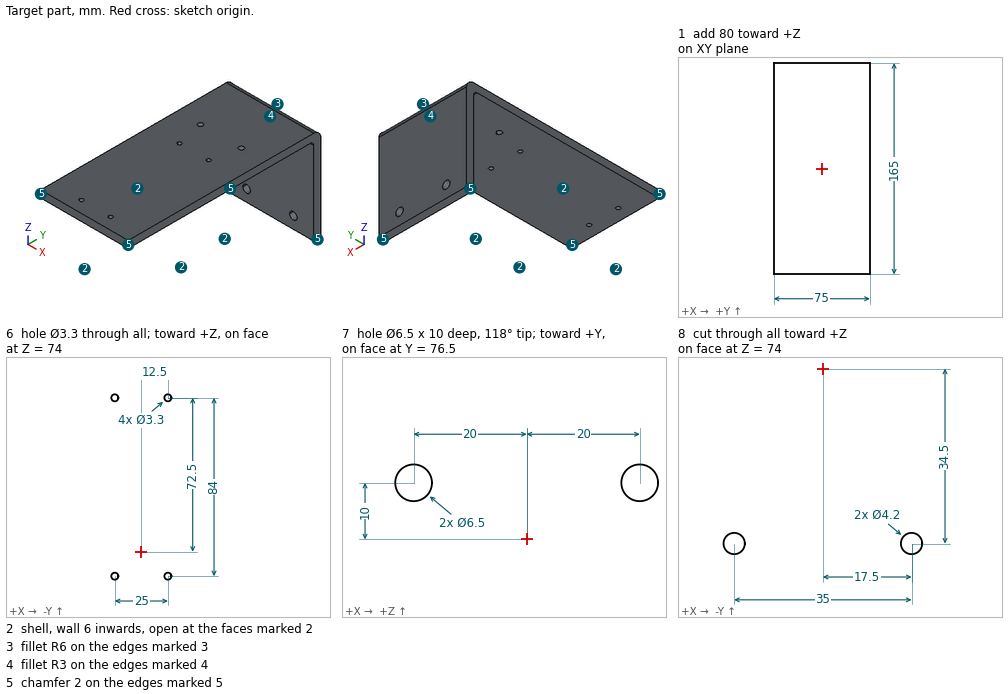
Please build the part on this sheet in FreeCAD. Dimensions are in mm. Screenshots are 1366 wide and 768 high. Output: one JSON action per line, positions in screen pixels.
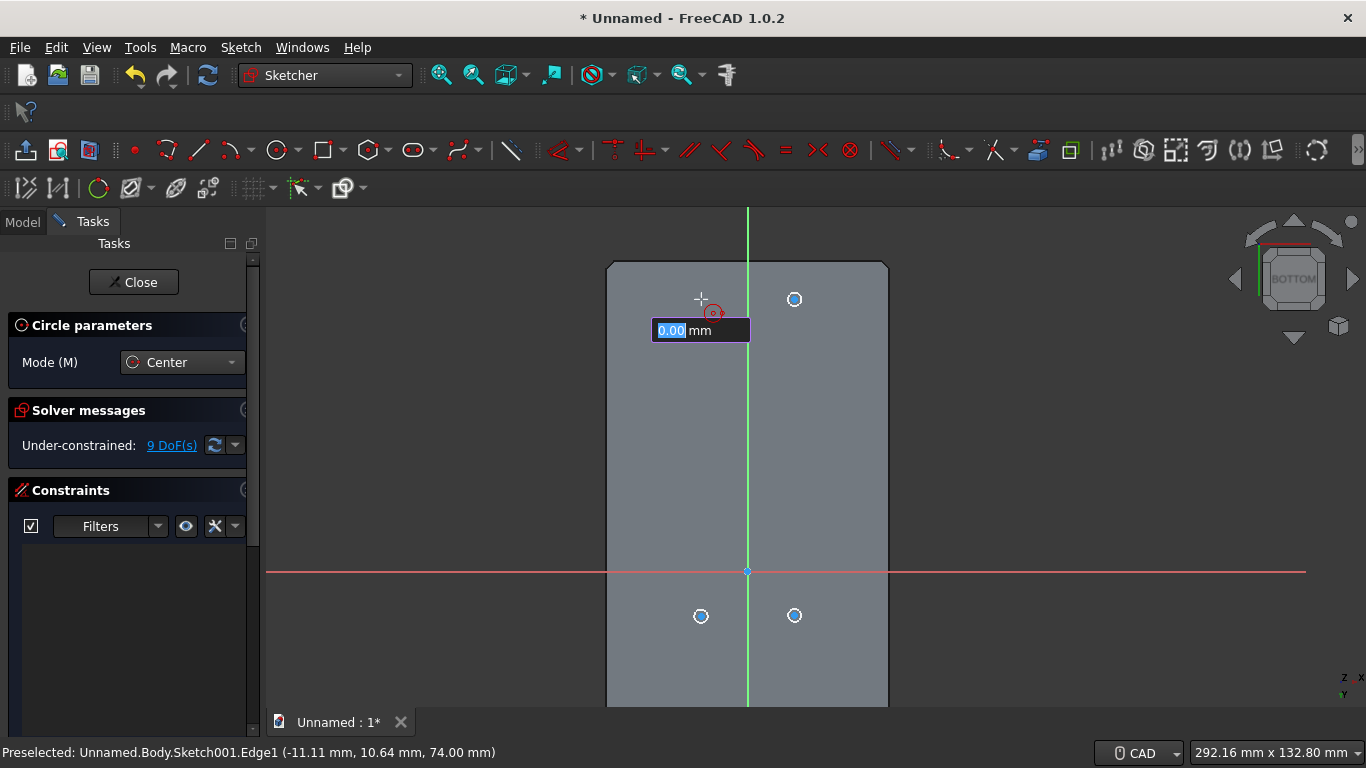
{"action": "scroll", "coordinate": [705, 294], "scroll_direction": "up", "scroll_amount": 5}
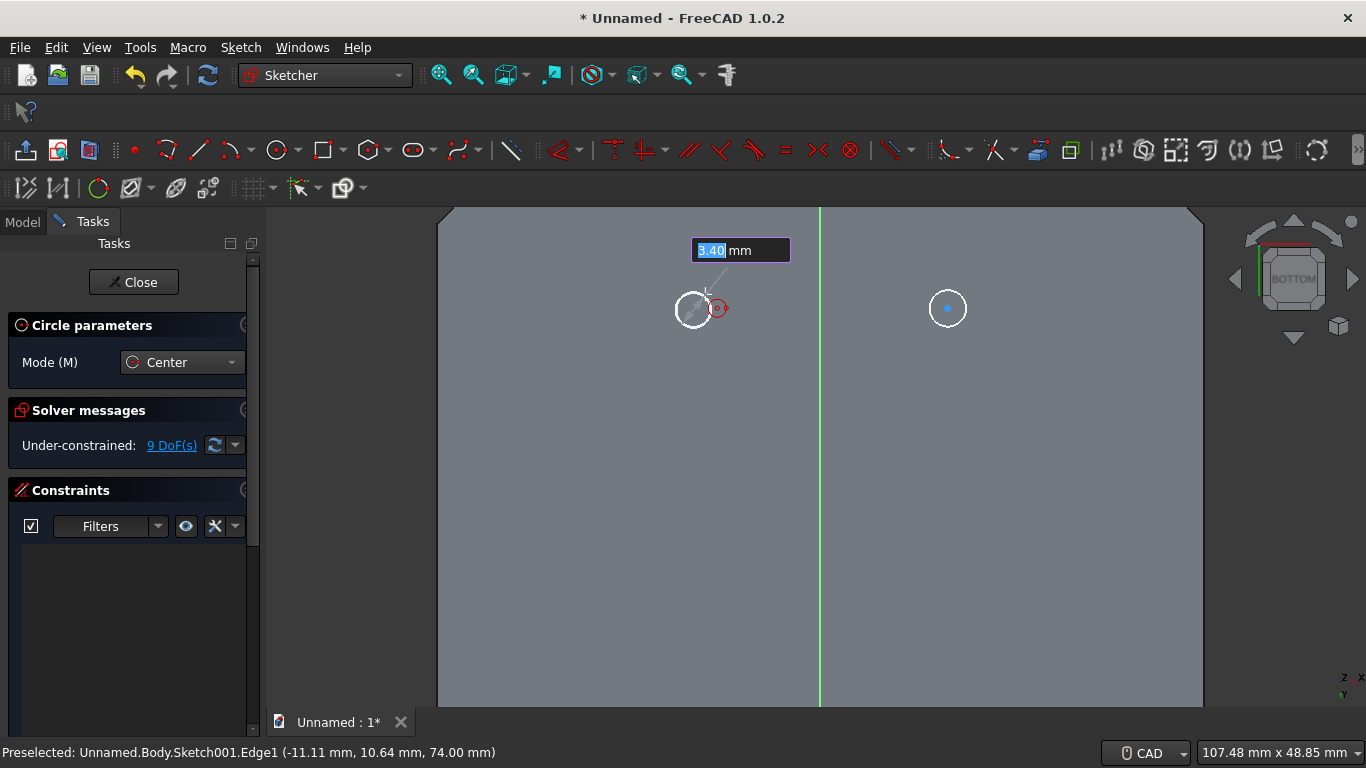
{"action": "left_click", "coordinate": [704, 294]}
{"action": "key", "text": "Escape"}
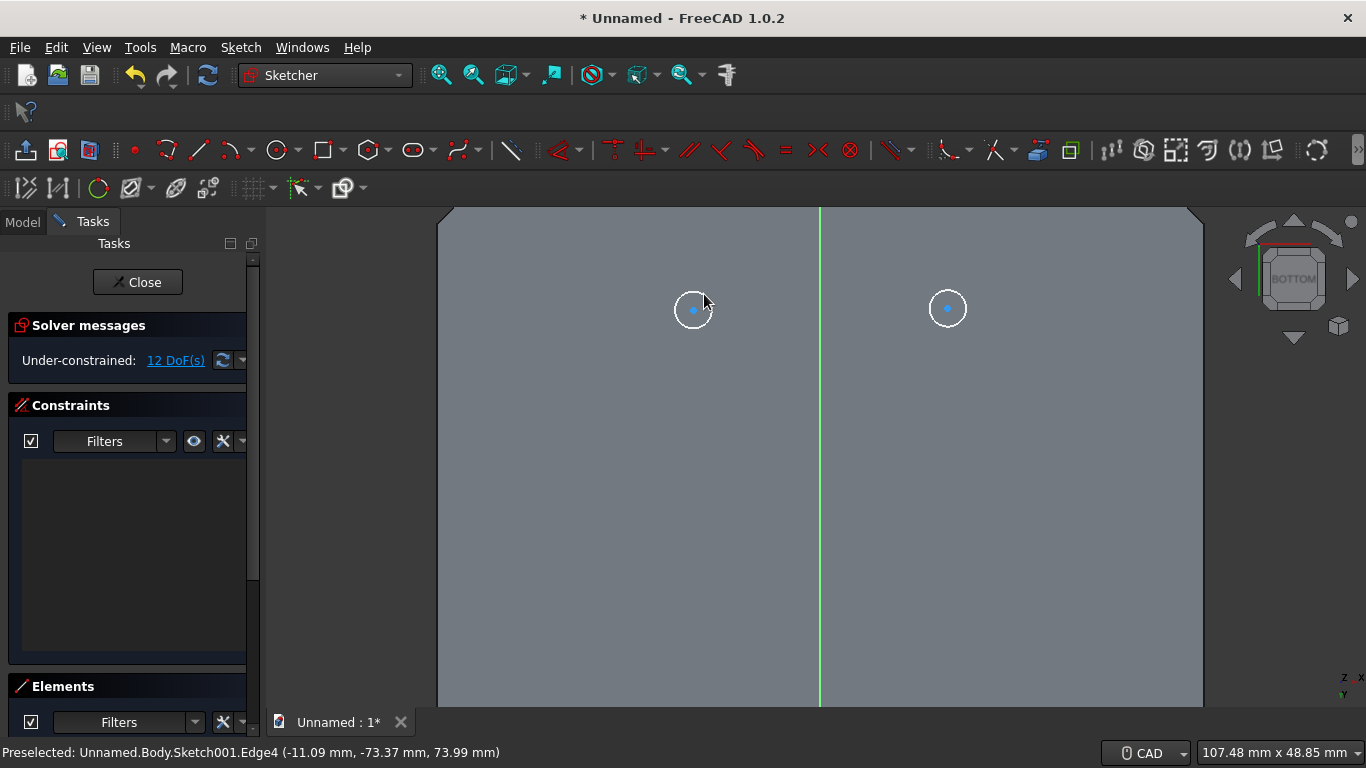
{"action": "left_click", "coordinate": [961, 296]}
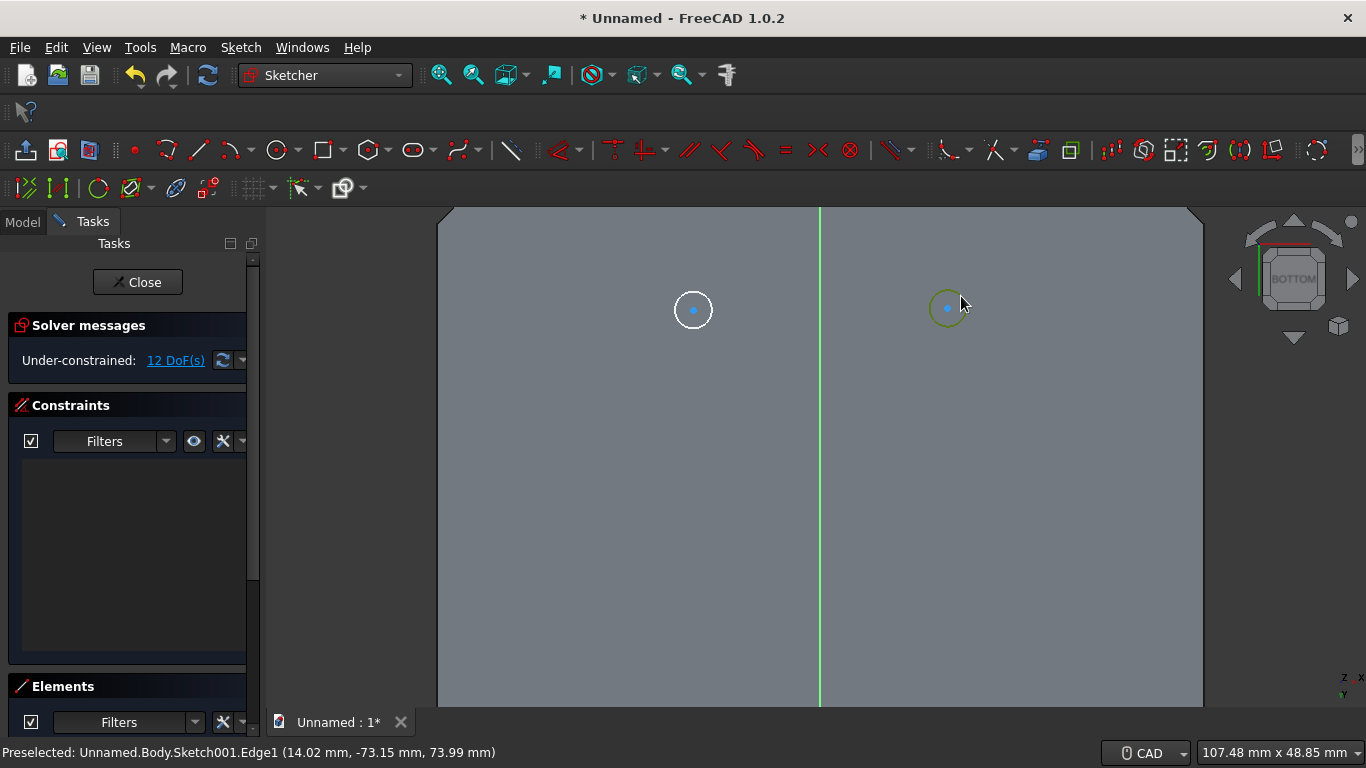
{"action": "scroll", "coordinate": [705, 295], "scroll_direction": "down", "scroll_amount": 5}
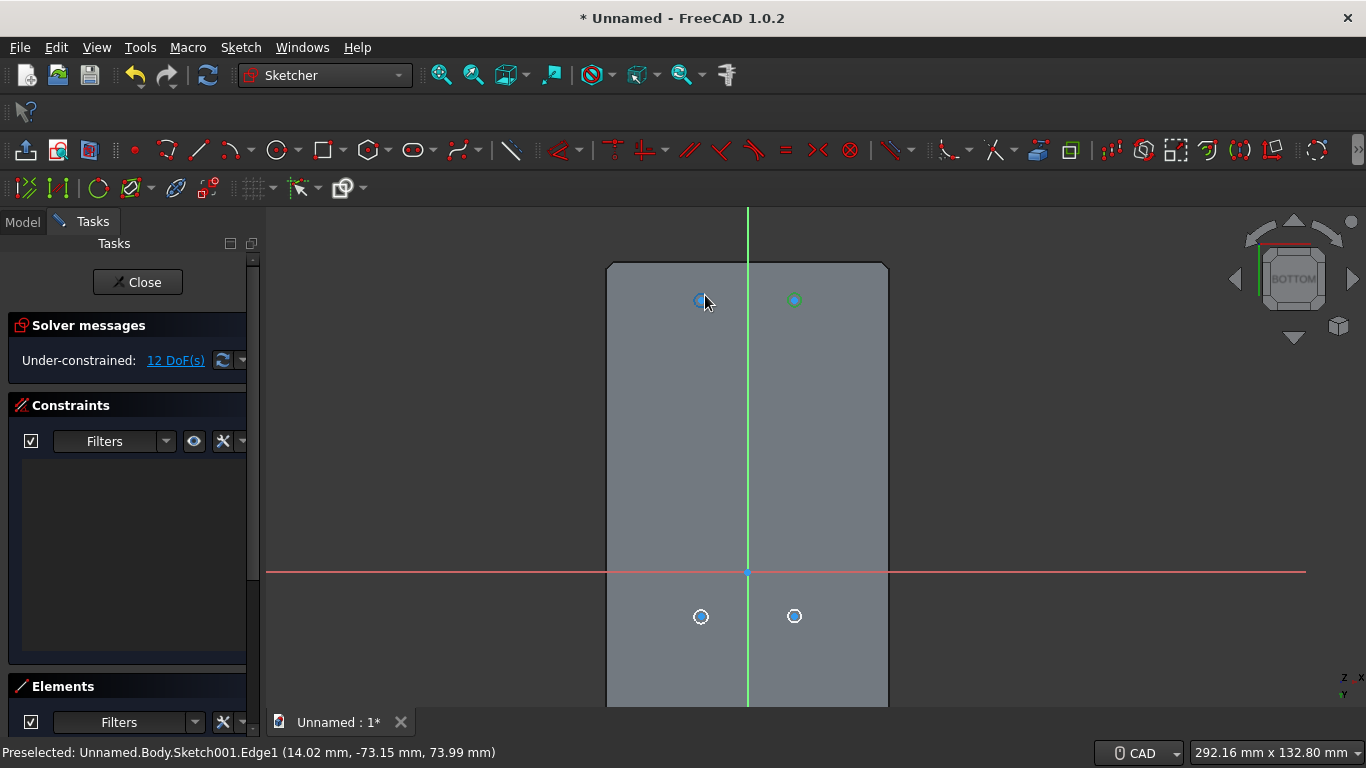
{"action": "scroll", "coordinate": [799, 612], "scroll_direction": "up", "scroll_amount": 4}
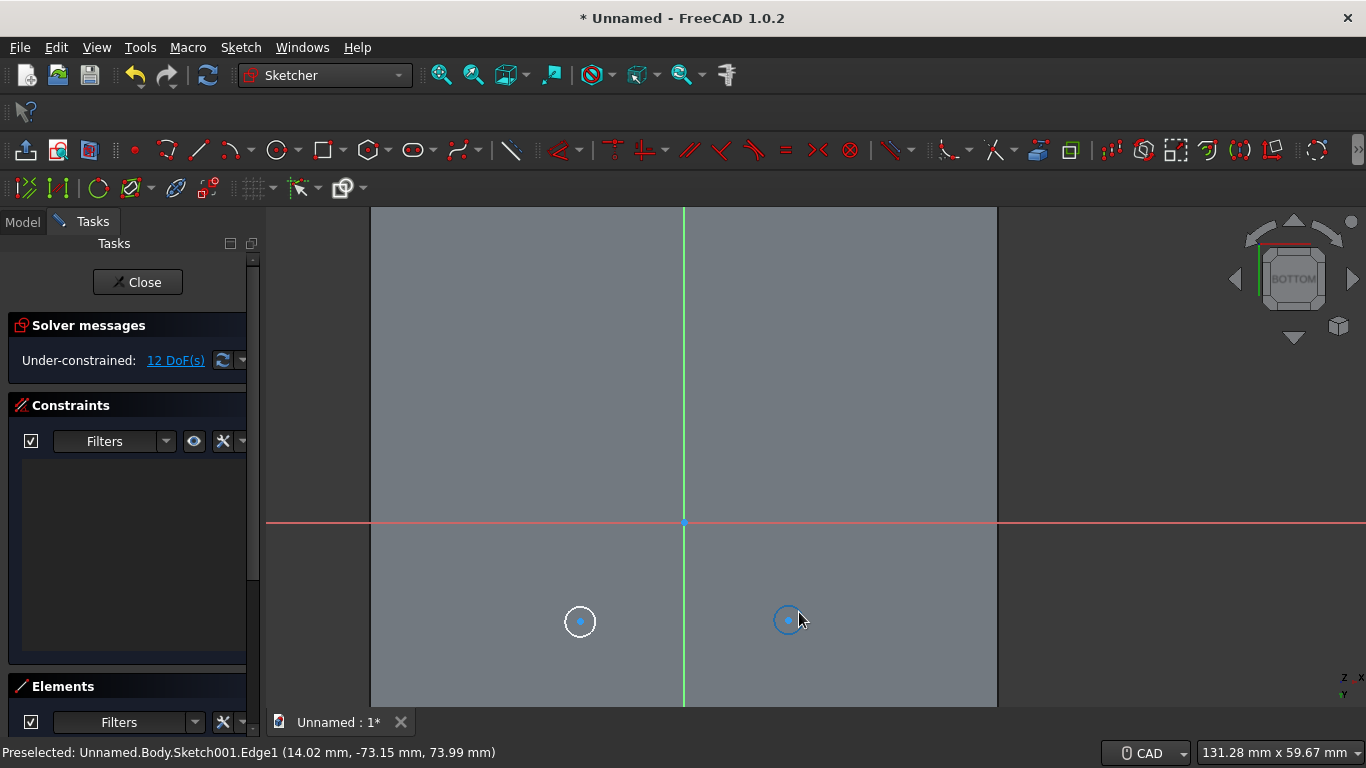
{"action": "left_click", "coordinate": [799, 610]}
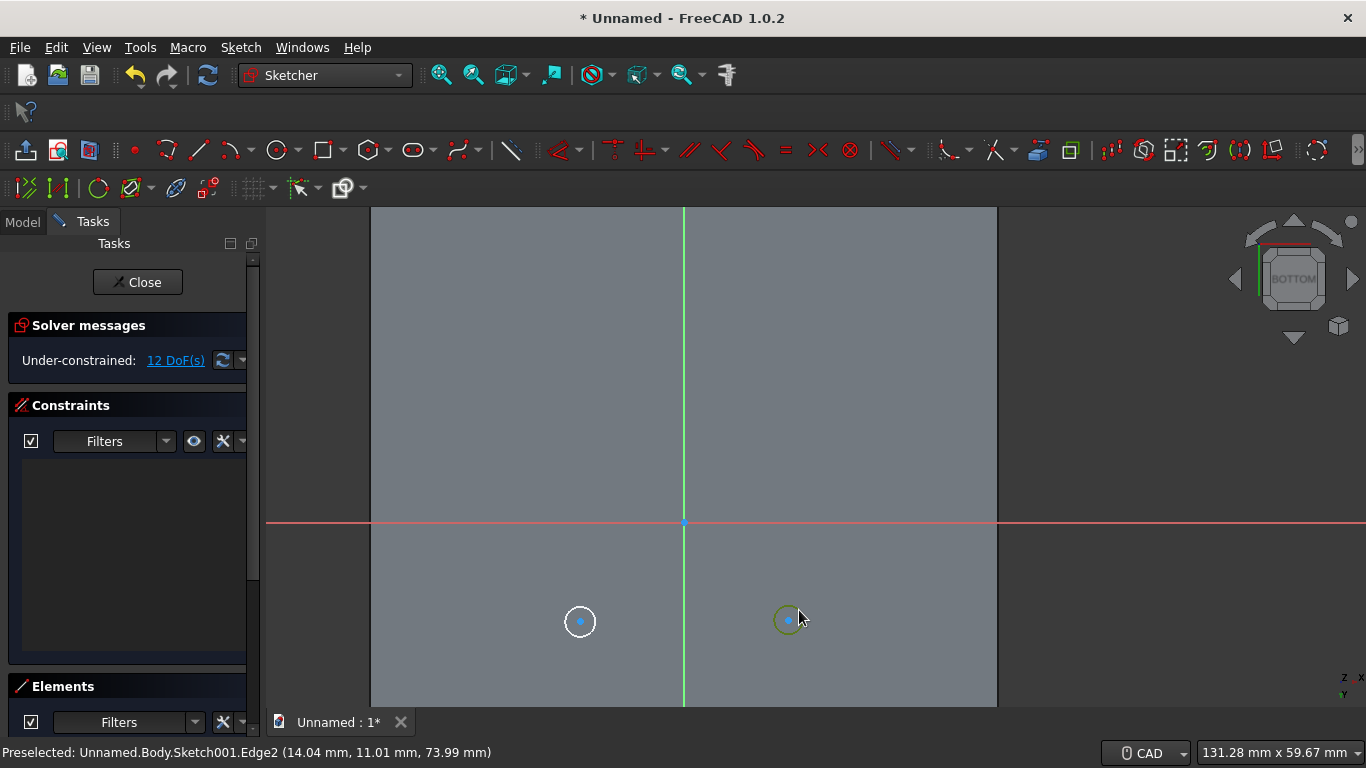
{"action": "left_click", "coordinate": [591, 611]}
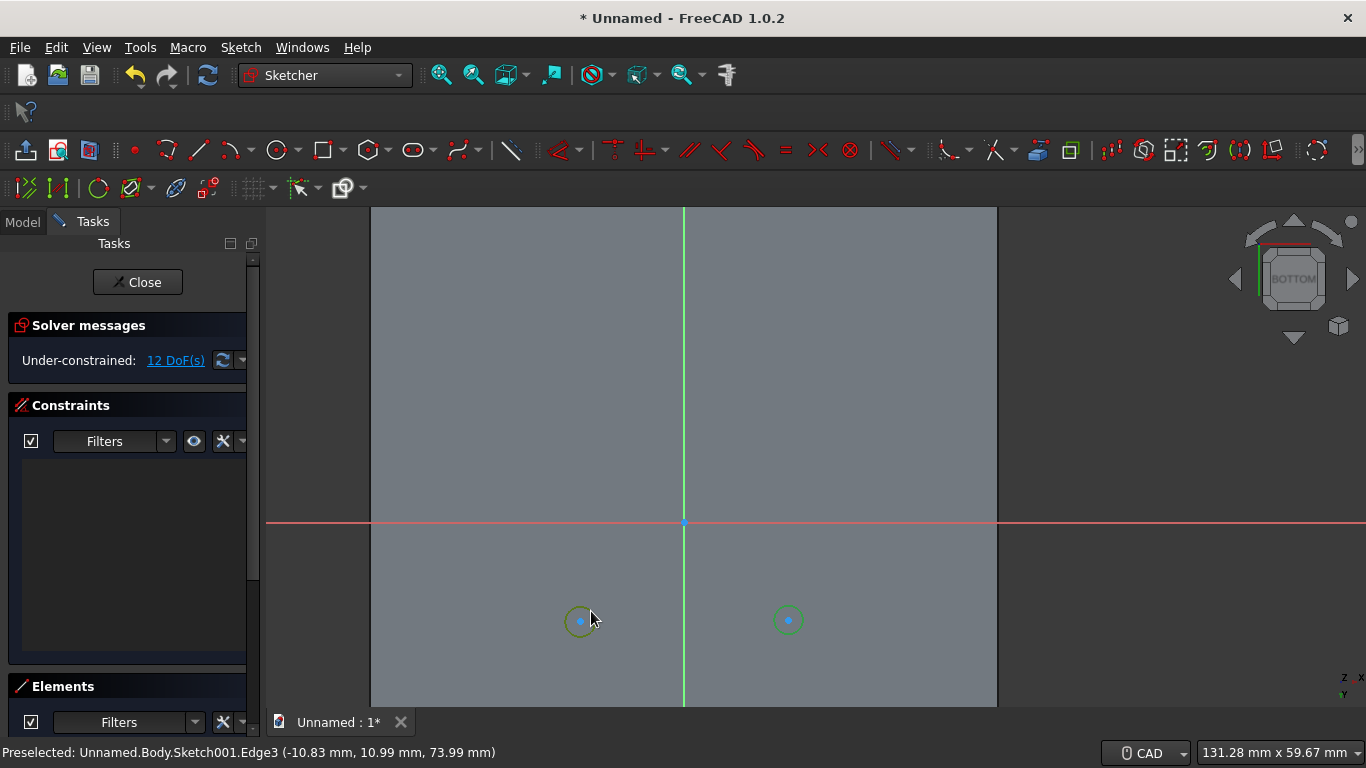
{"action": "scroll", "coordinate": [799, 612], "scroll_direction": "down", "scroll_amount": 4}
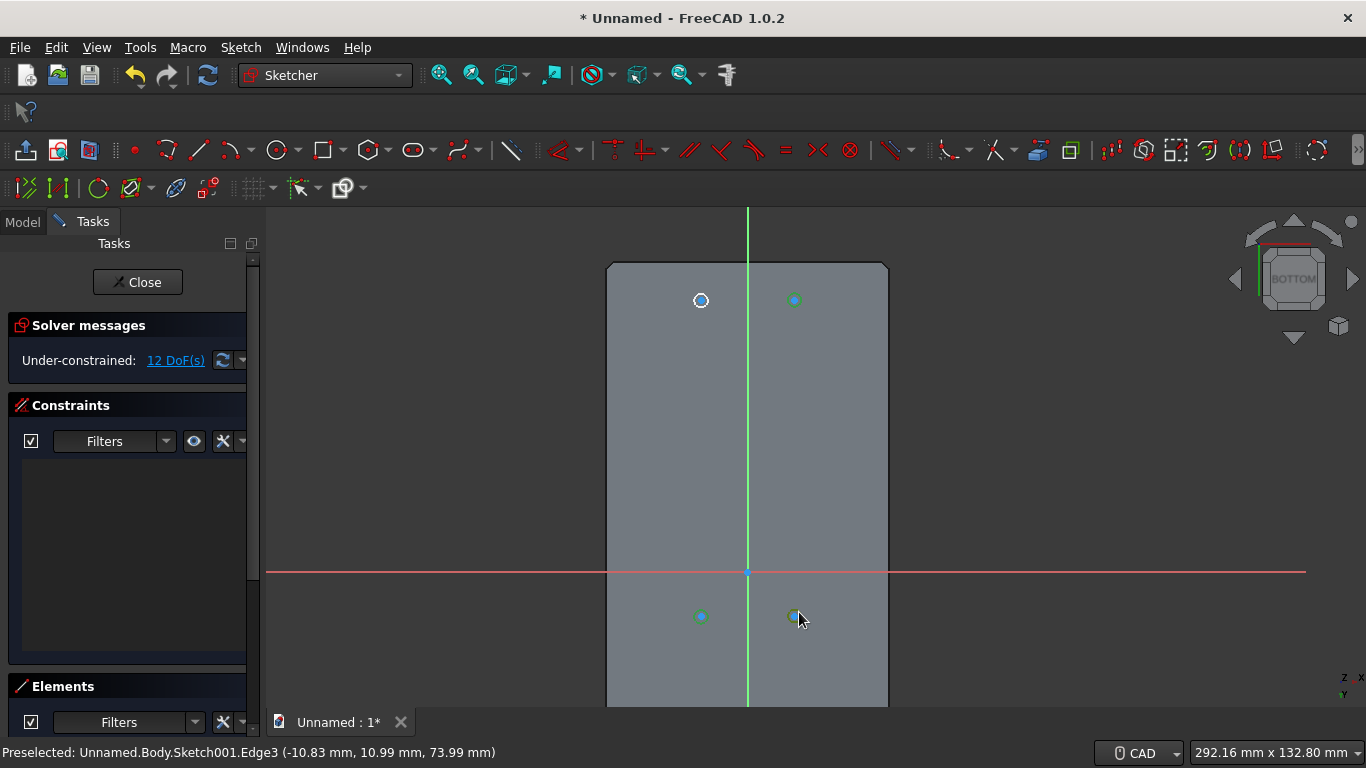
{"action": "scroll", "coordinate": [706, 296], "scroll_direction": "up", "scroll_amount": 4}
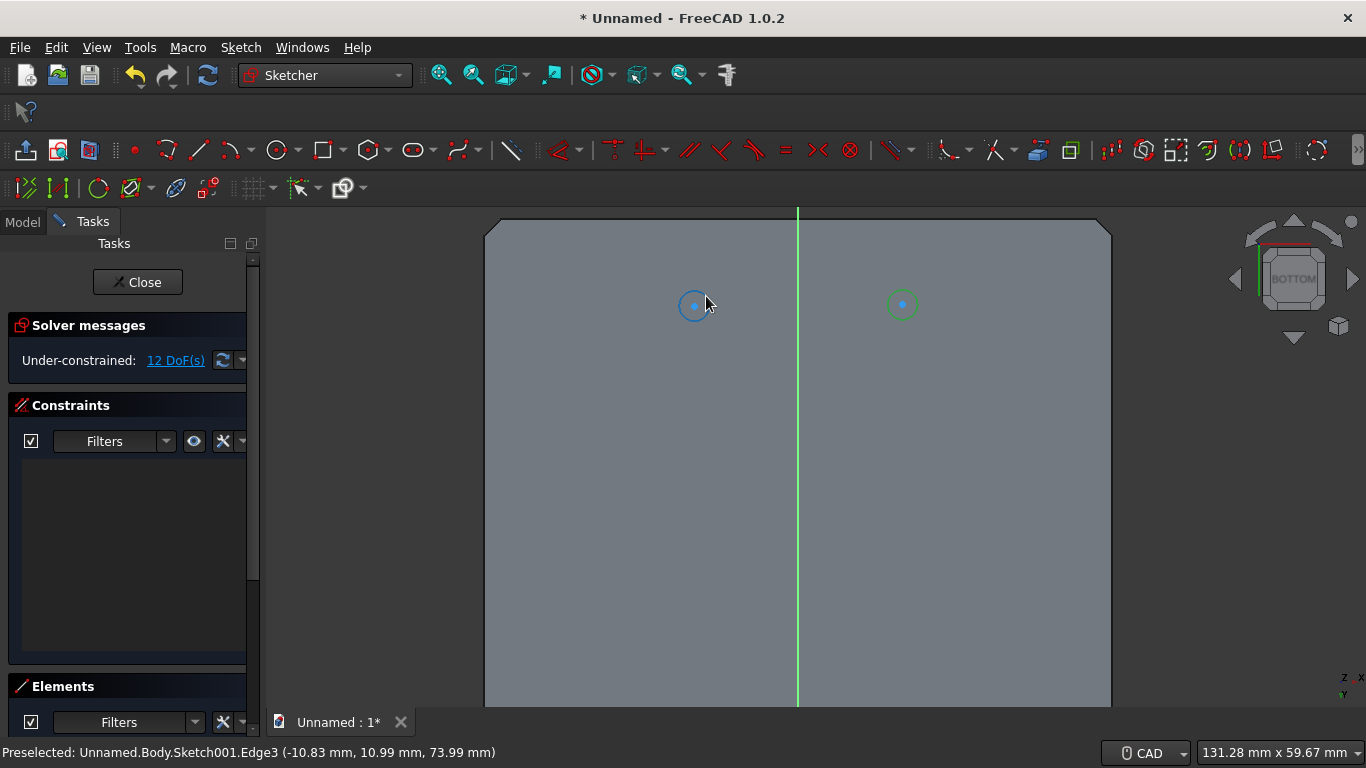
{"action": "left_click", "coordinate": [705, 295]}